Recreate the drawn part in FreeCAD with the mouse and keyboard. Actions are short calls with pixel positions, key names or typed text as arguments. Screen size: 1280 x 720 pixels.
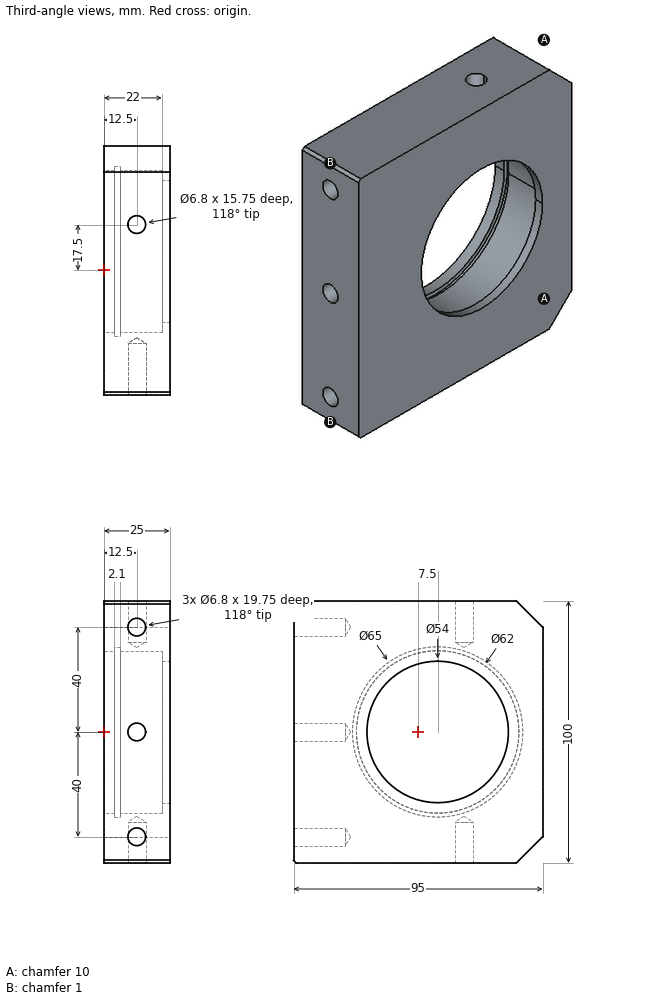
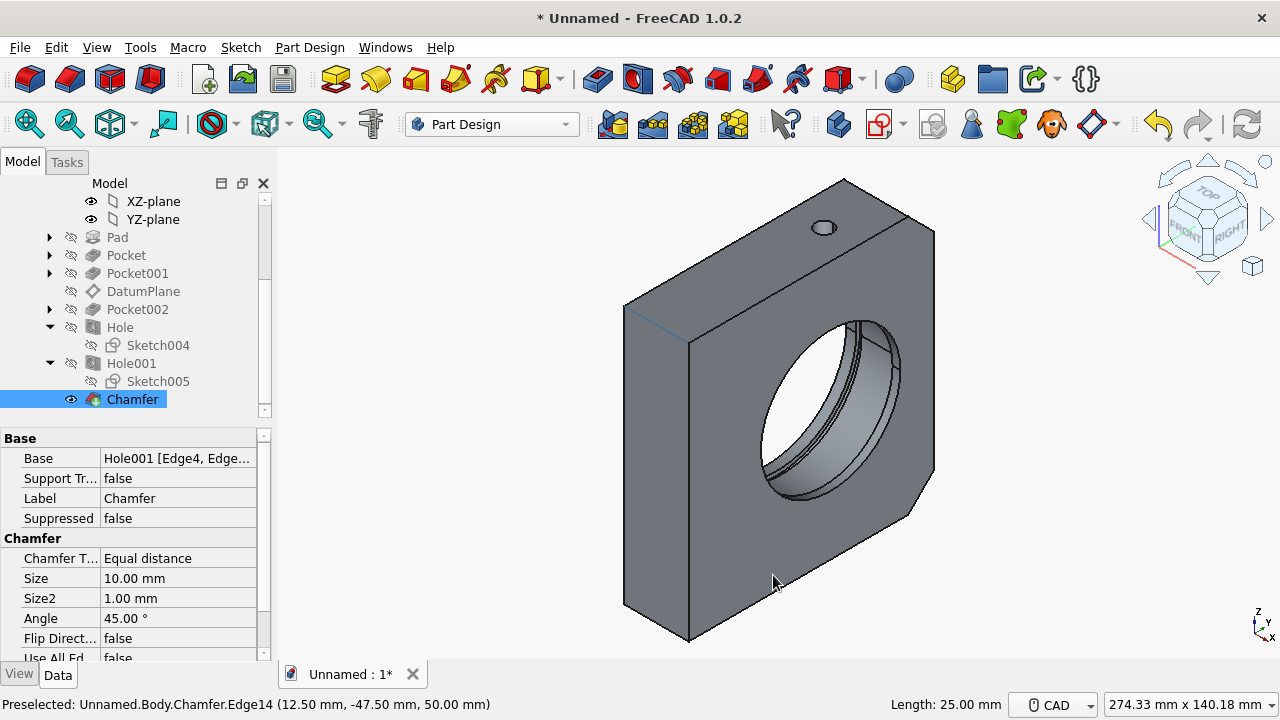
key(2)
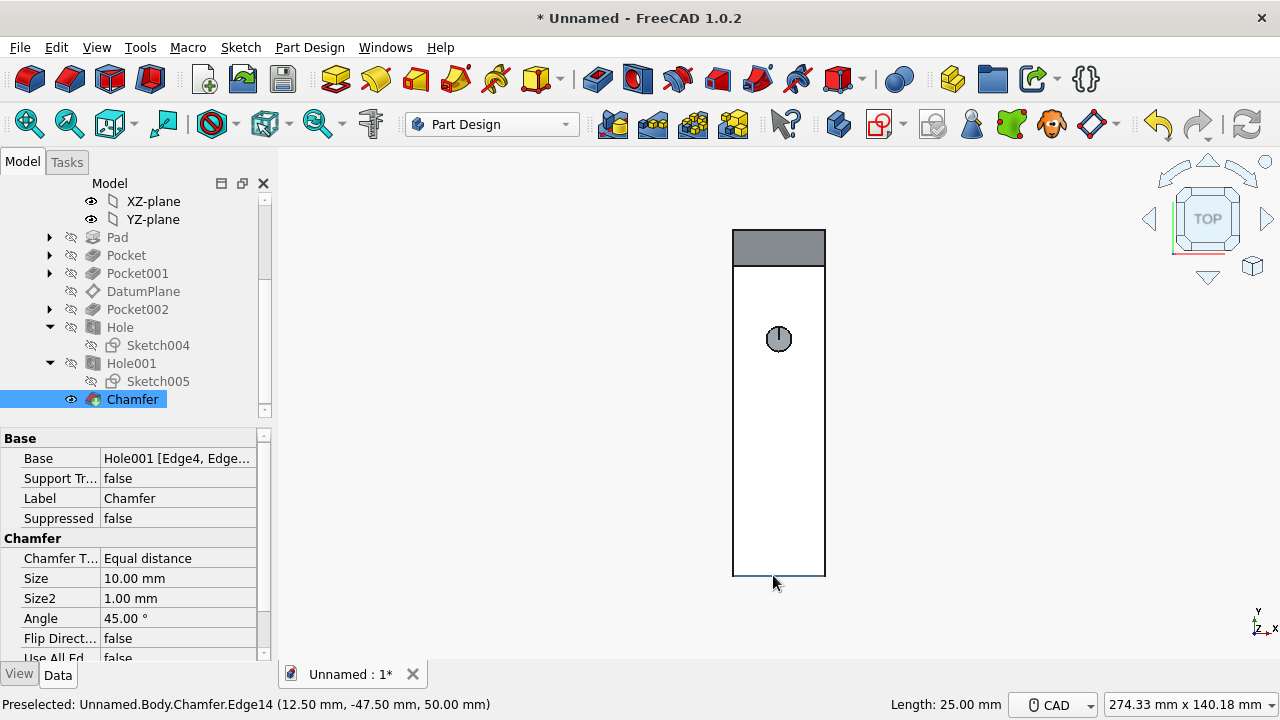
key(1)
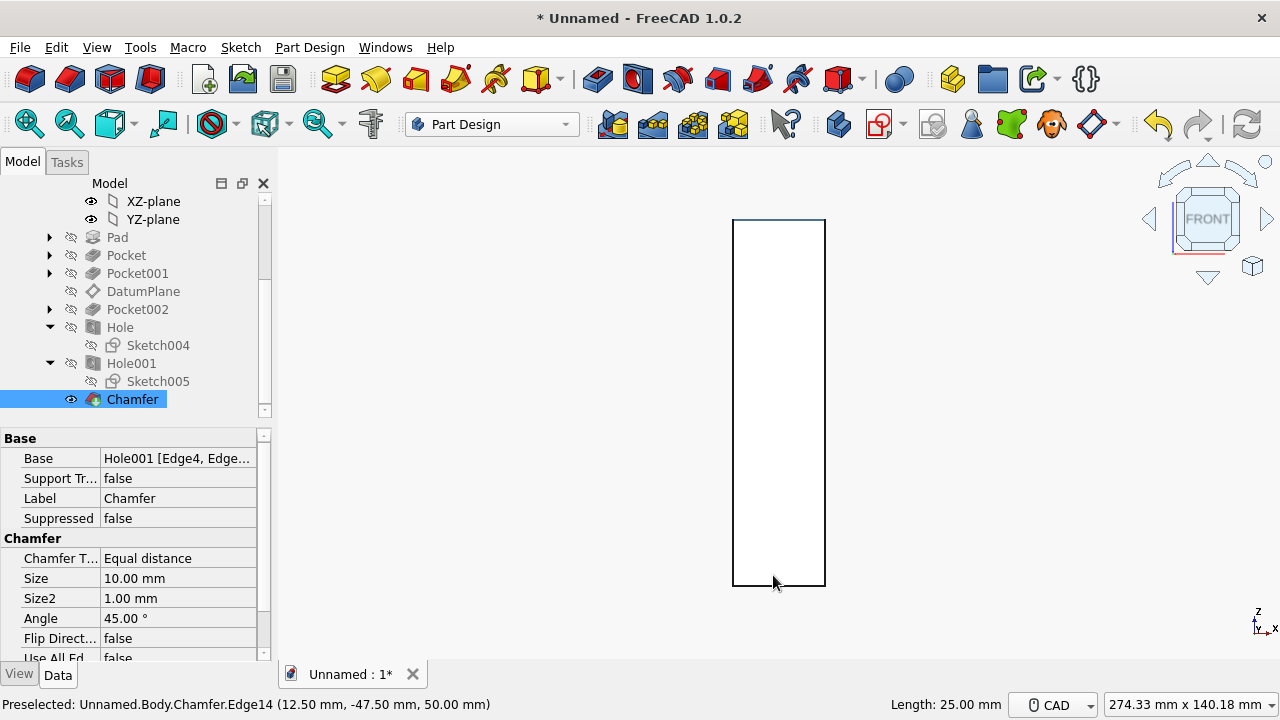
click(779, 585, ctrl)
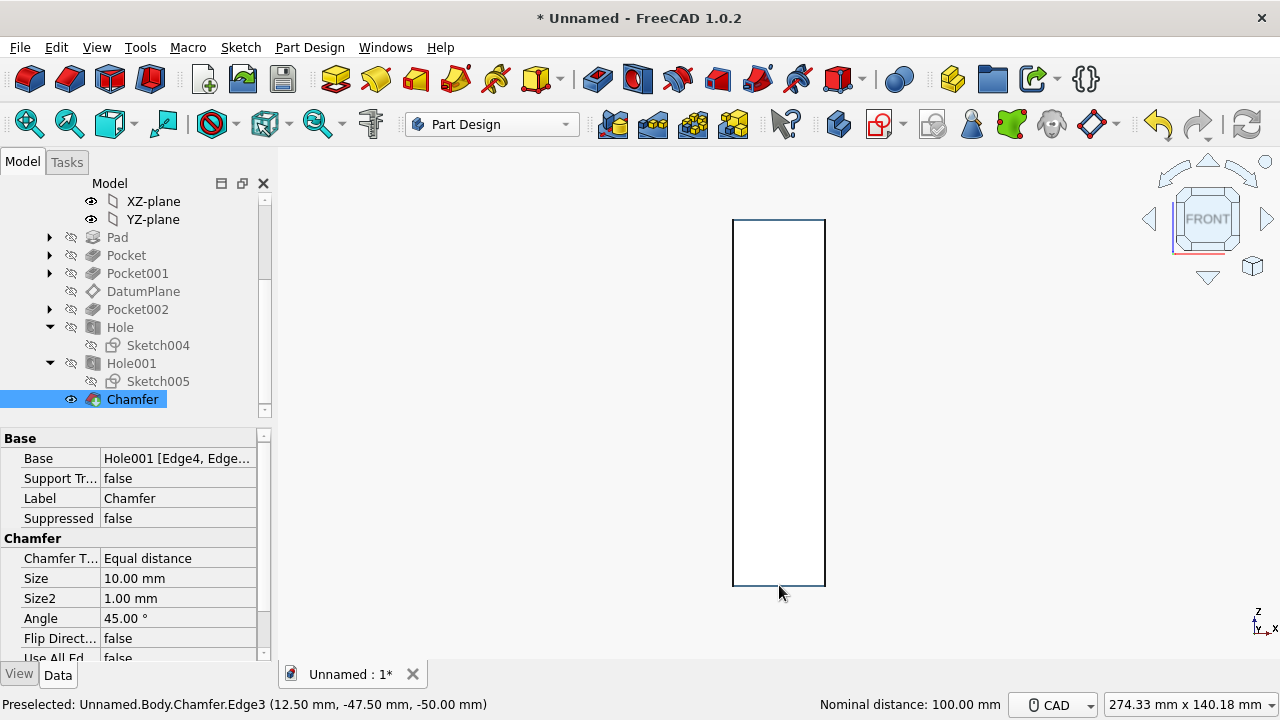
click(70, 80)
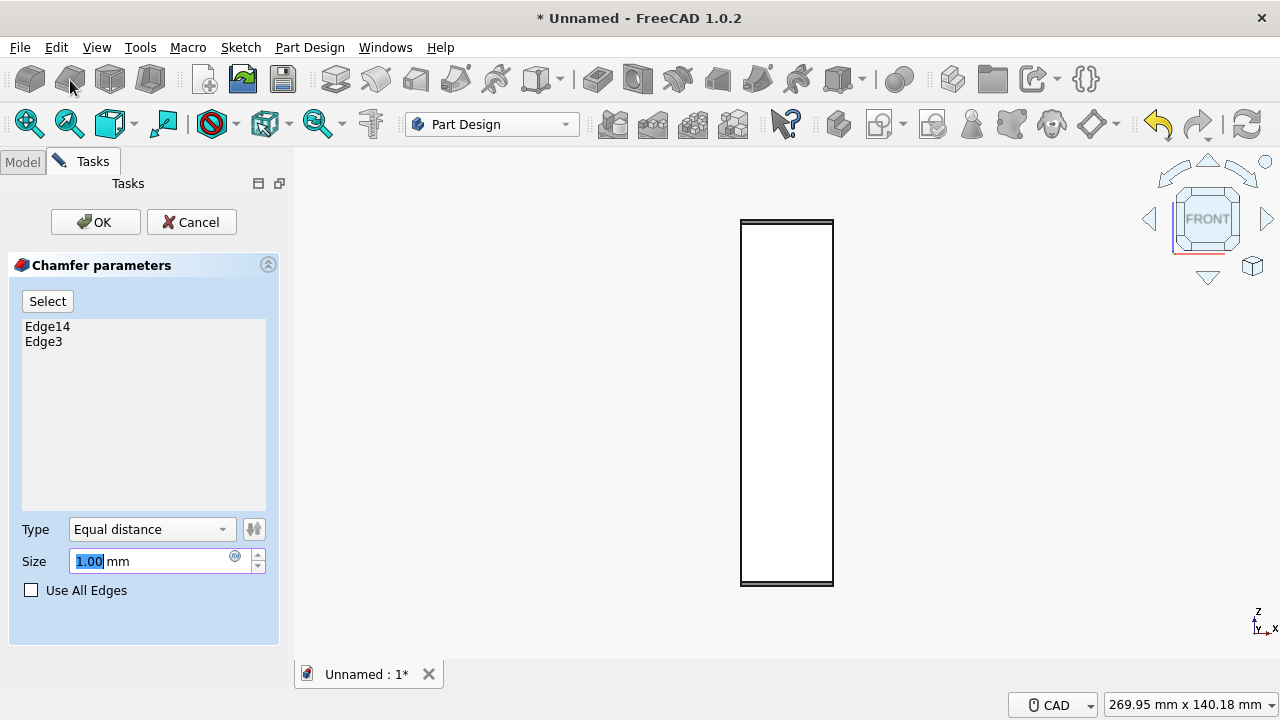
text(1)
key(Tab)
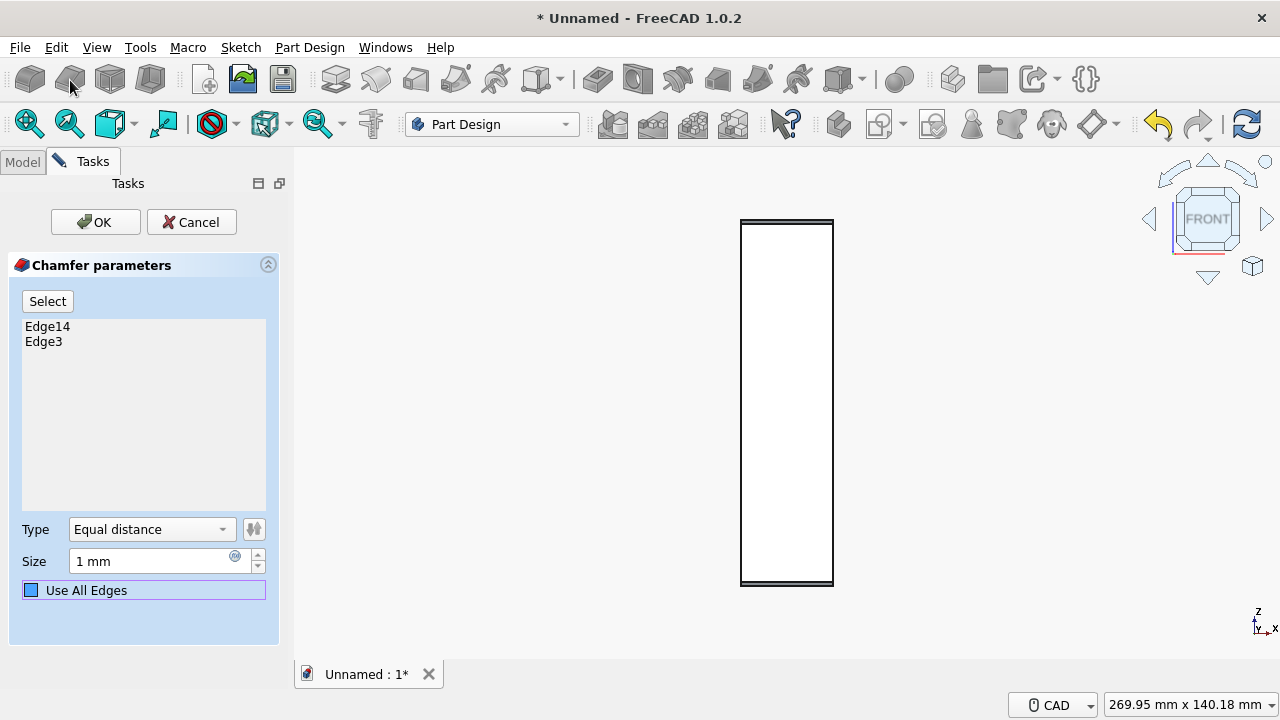
click(96, 222)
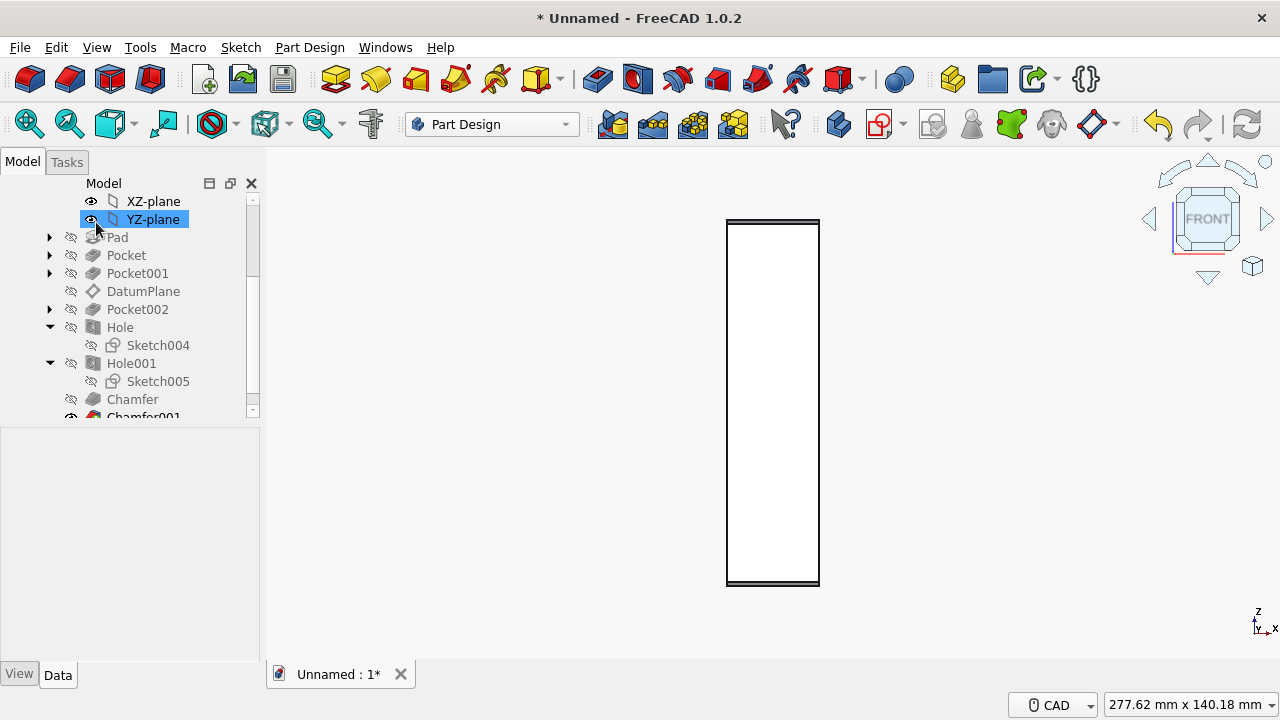
click(773, 504)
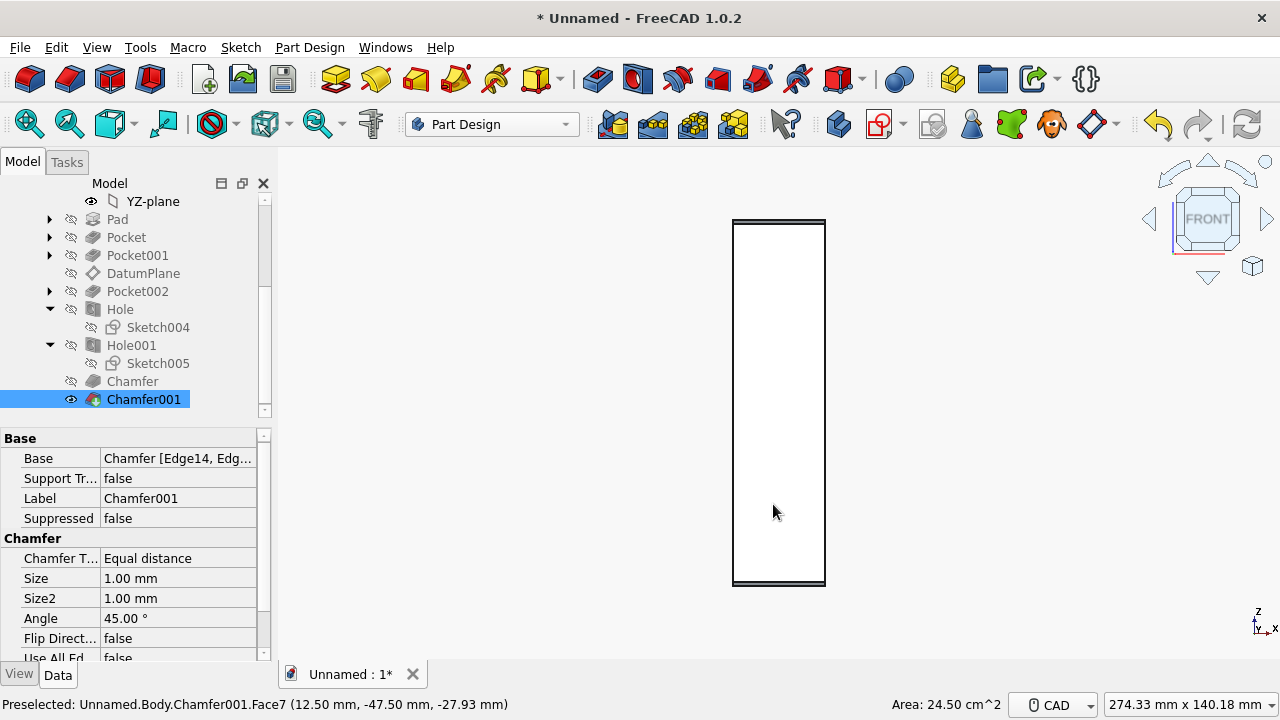
click(880, 124)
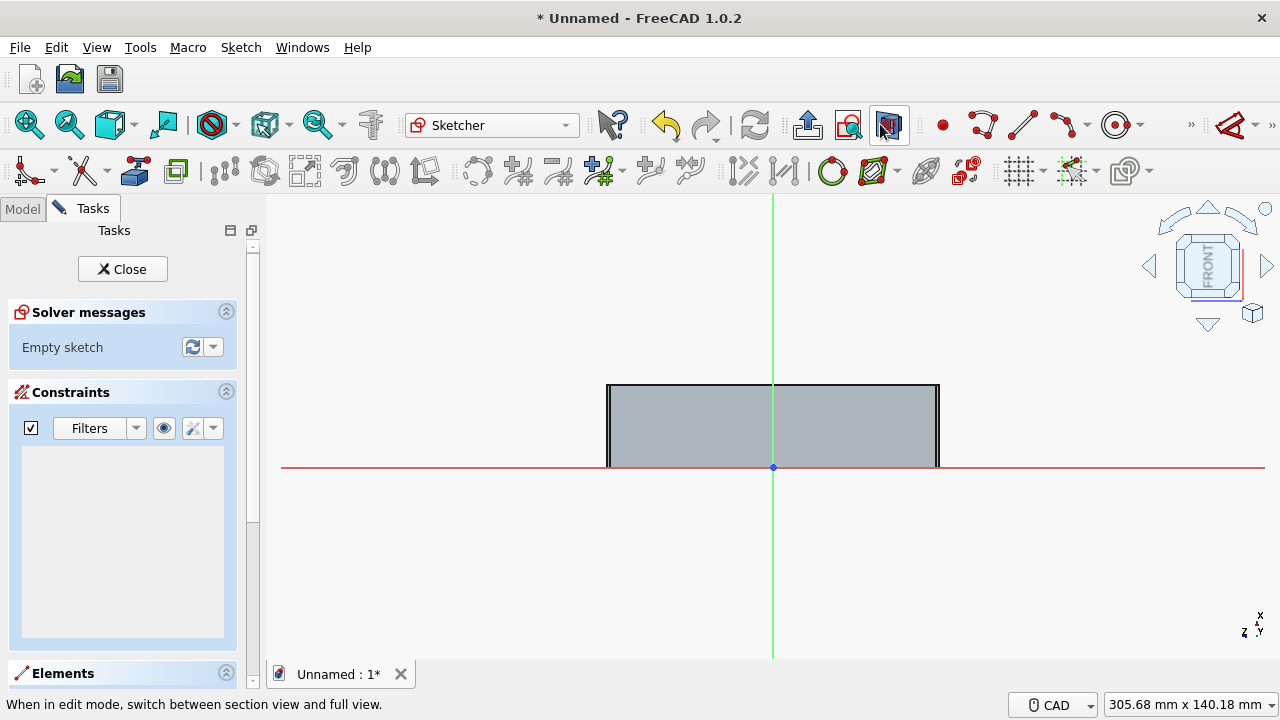
scroll(856, 460, up, 3)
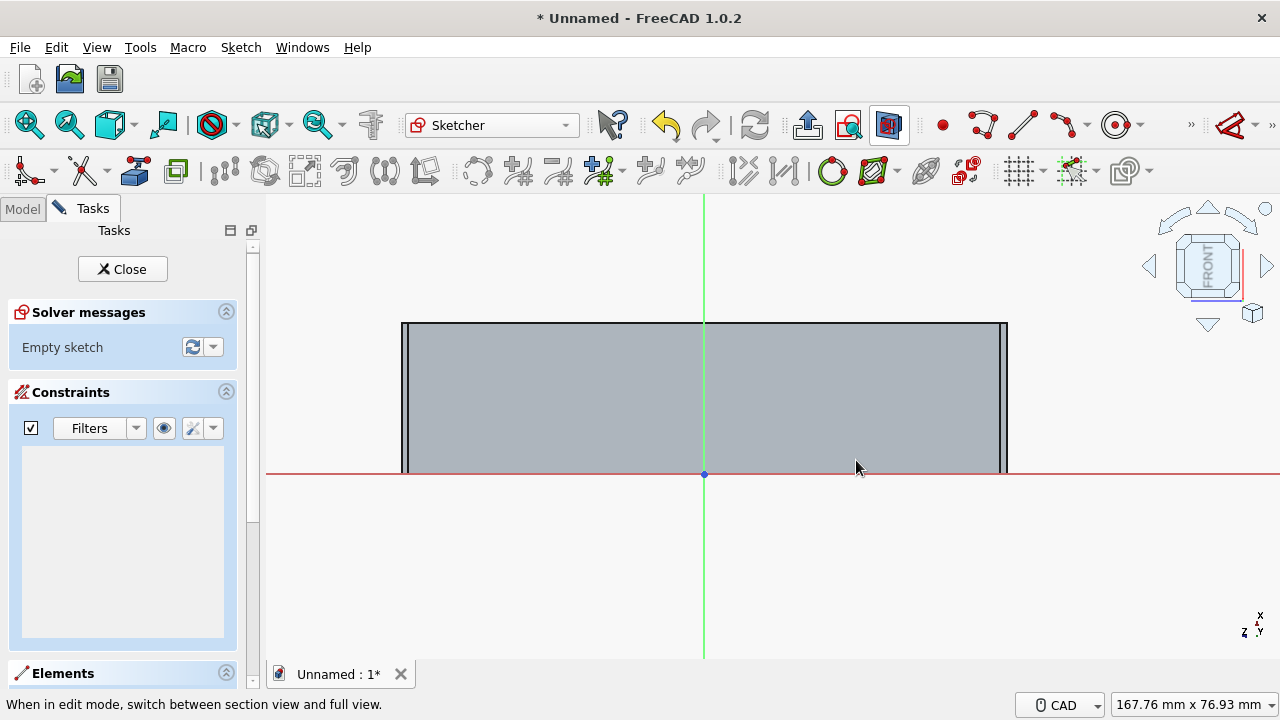
click(1116, 126)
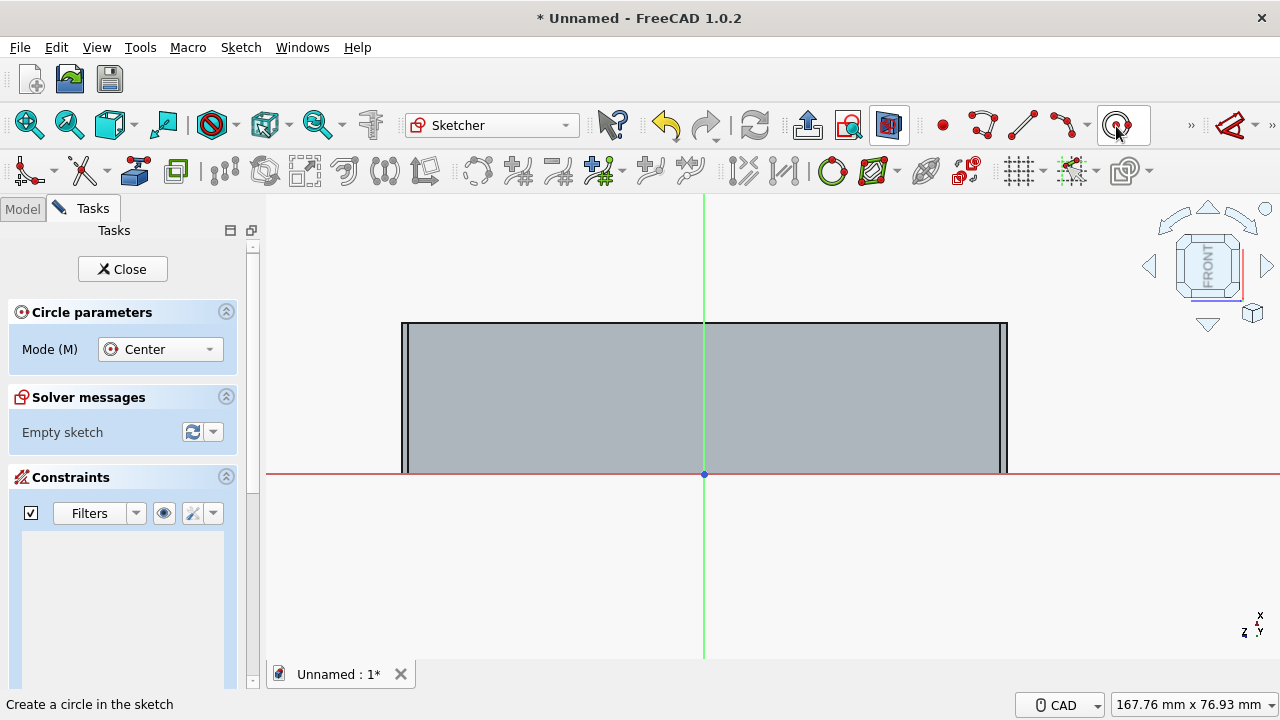
click(463, 398)
click(477, 384)